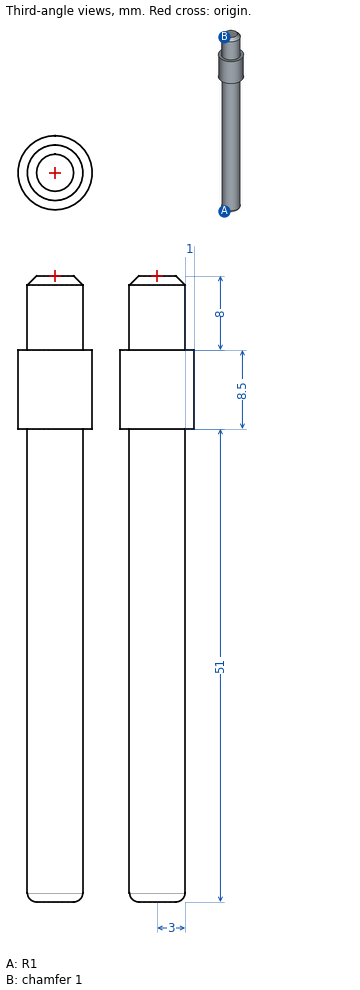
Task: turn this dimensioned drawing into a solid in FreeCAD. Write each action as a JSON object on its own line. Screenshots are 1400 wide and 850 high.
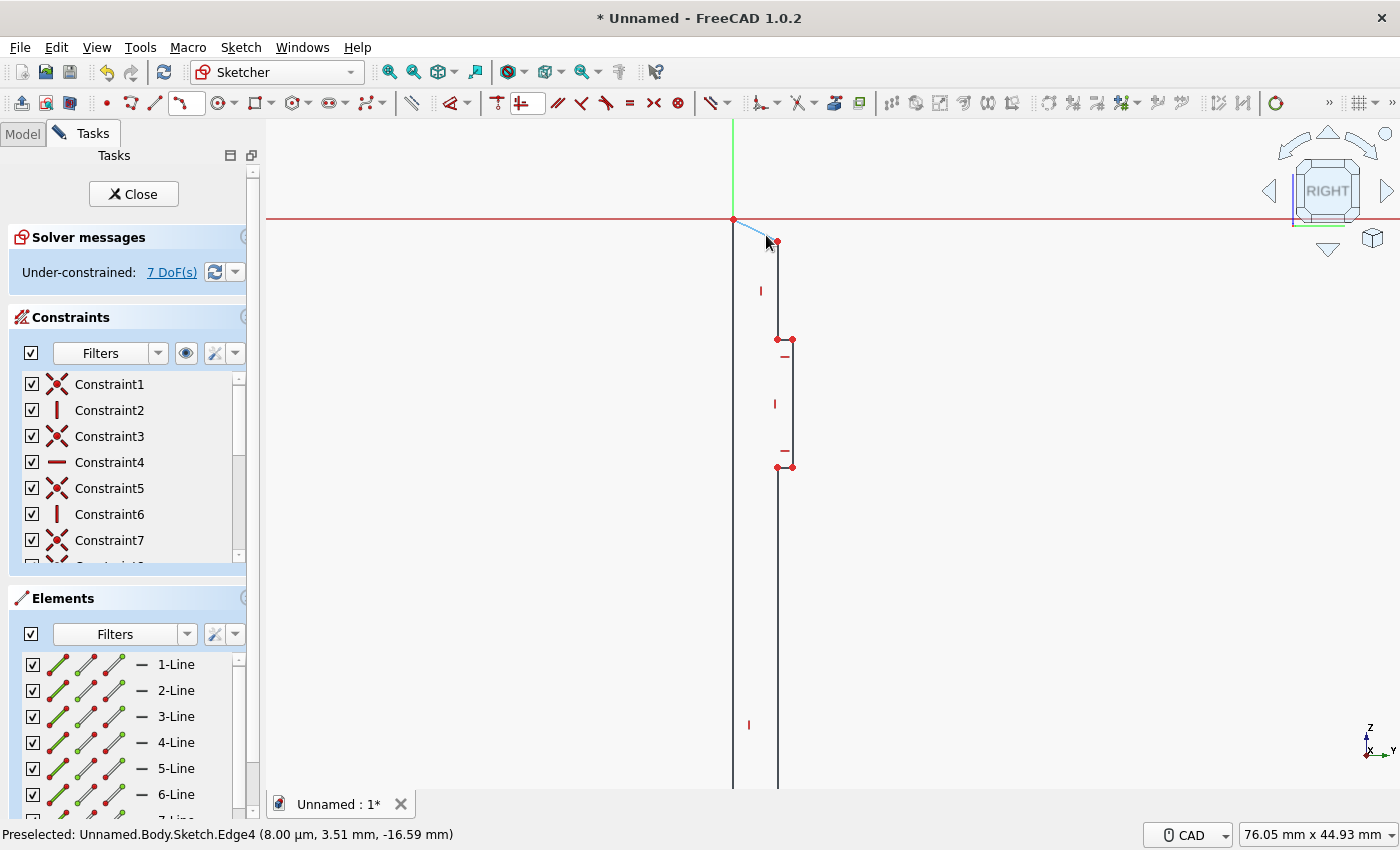
{"action": "left_click", "coordinate": [764, 235]}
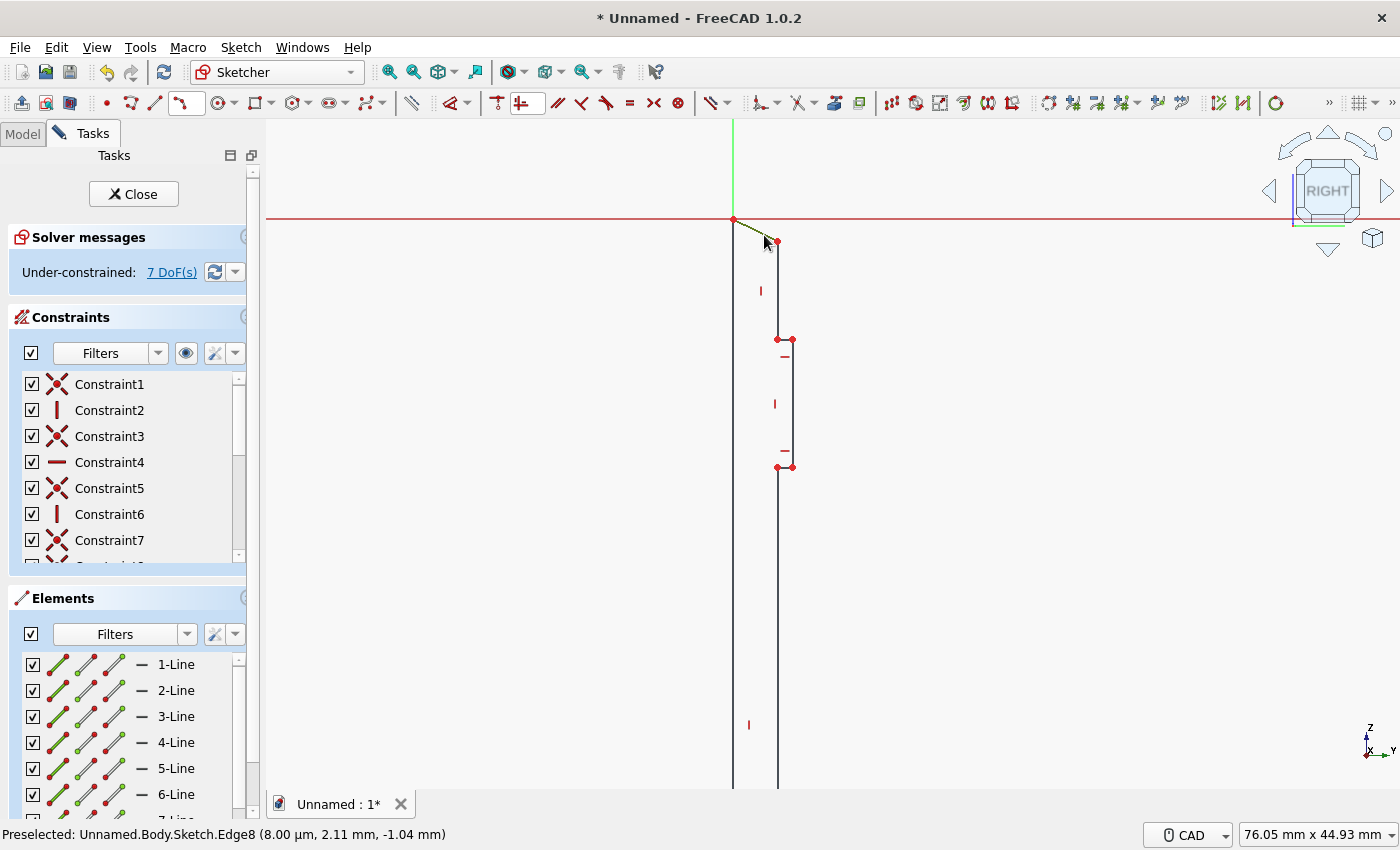
{"action": "key", "text": "h"}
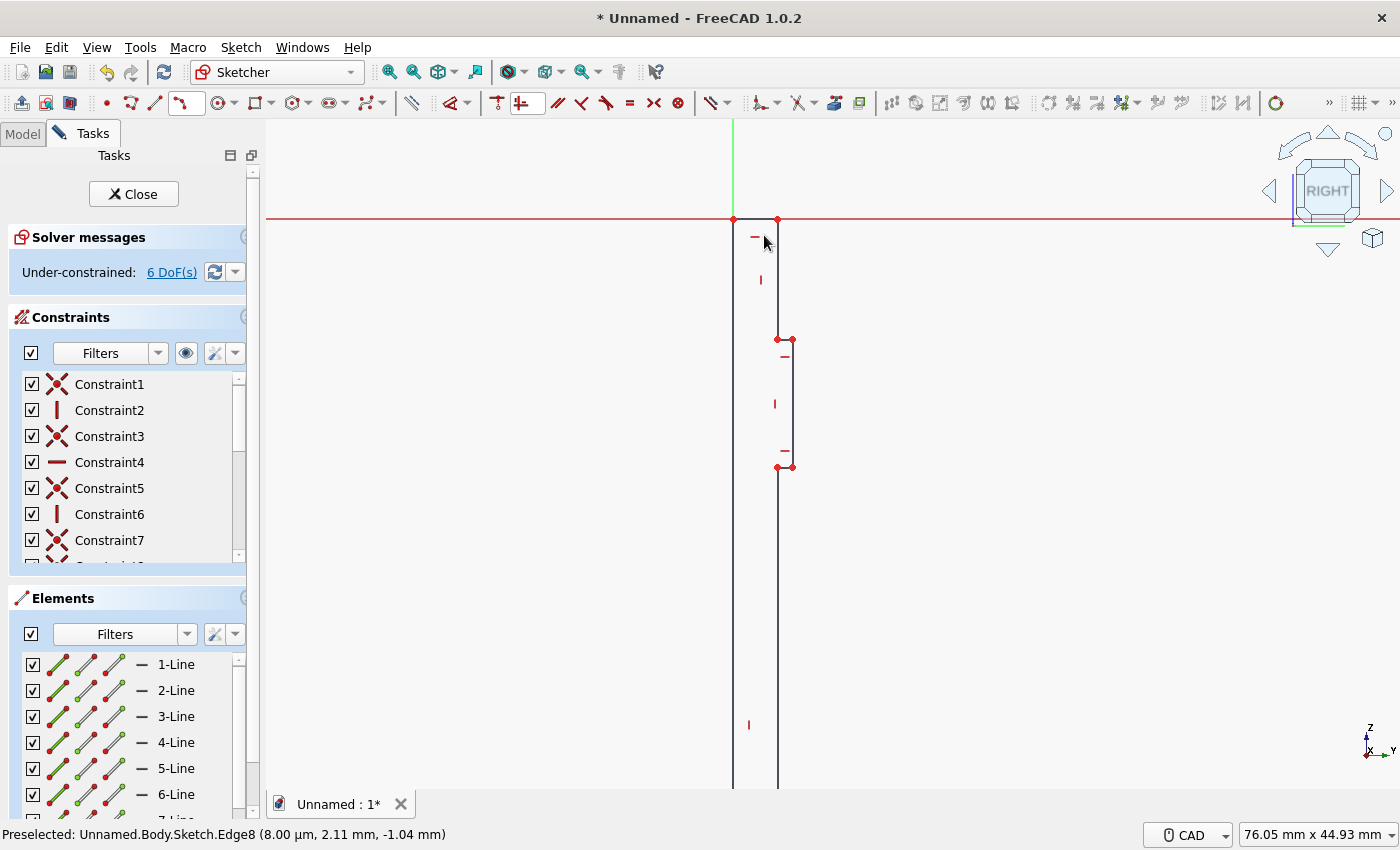
{"action": "key", "text": "d"}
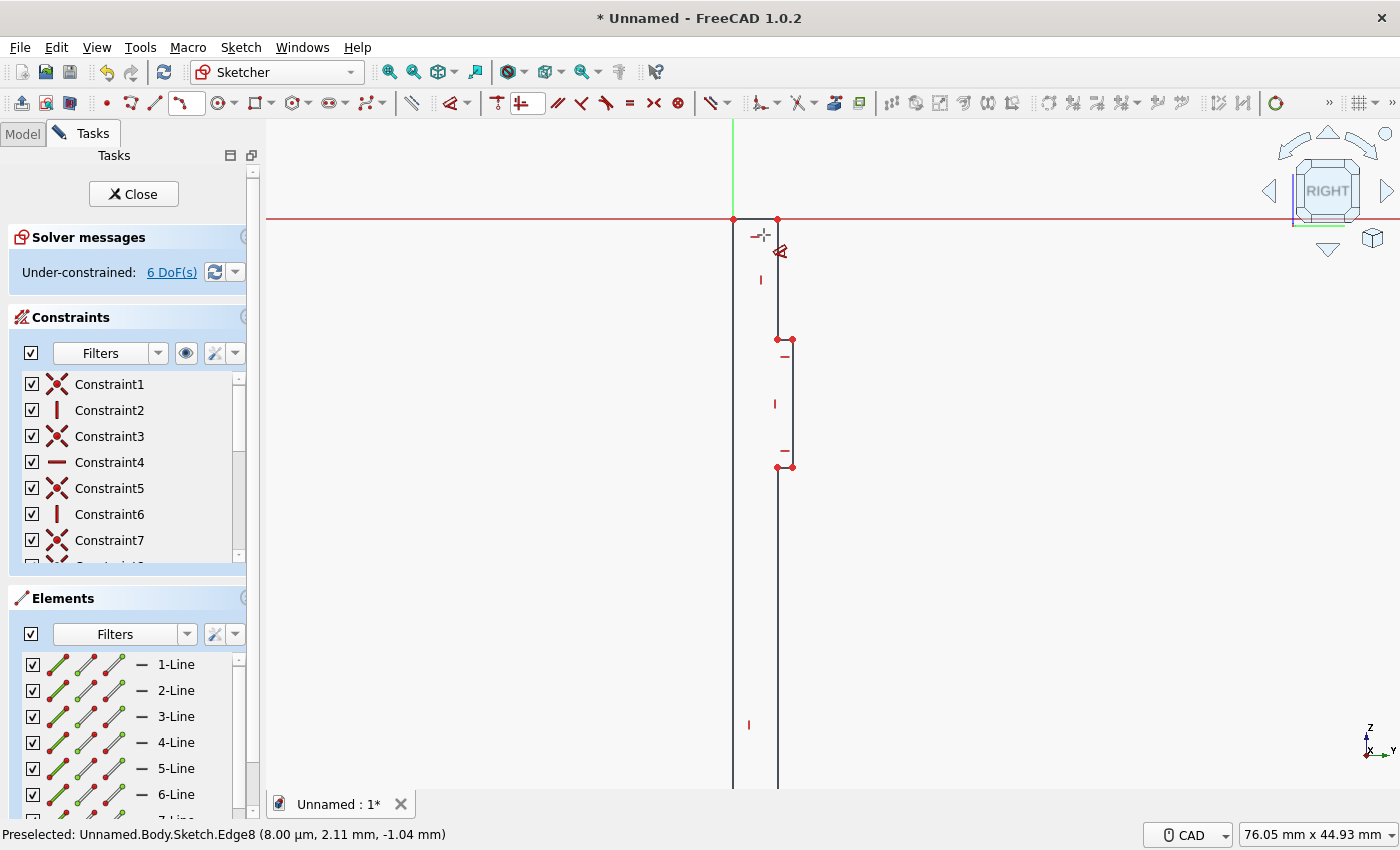
{"action": "scroll", "coordinate": [766, 235], "scroll_direction": "down", "scroll_amount": 4}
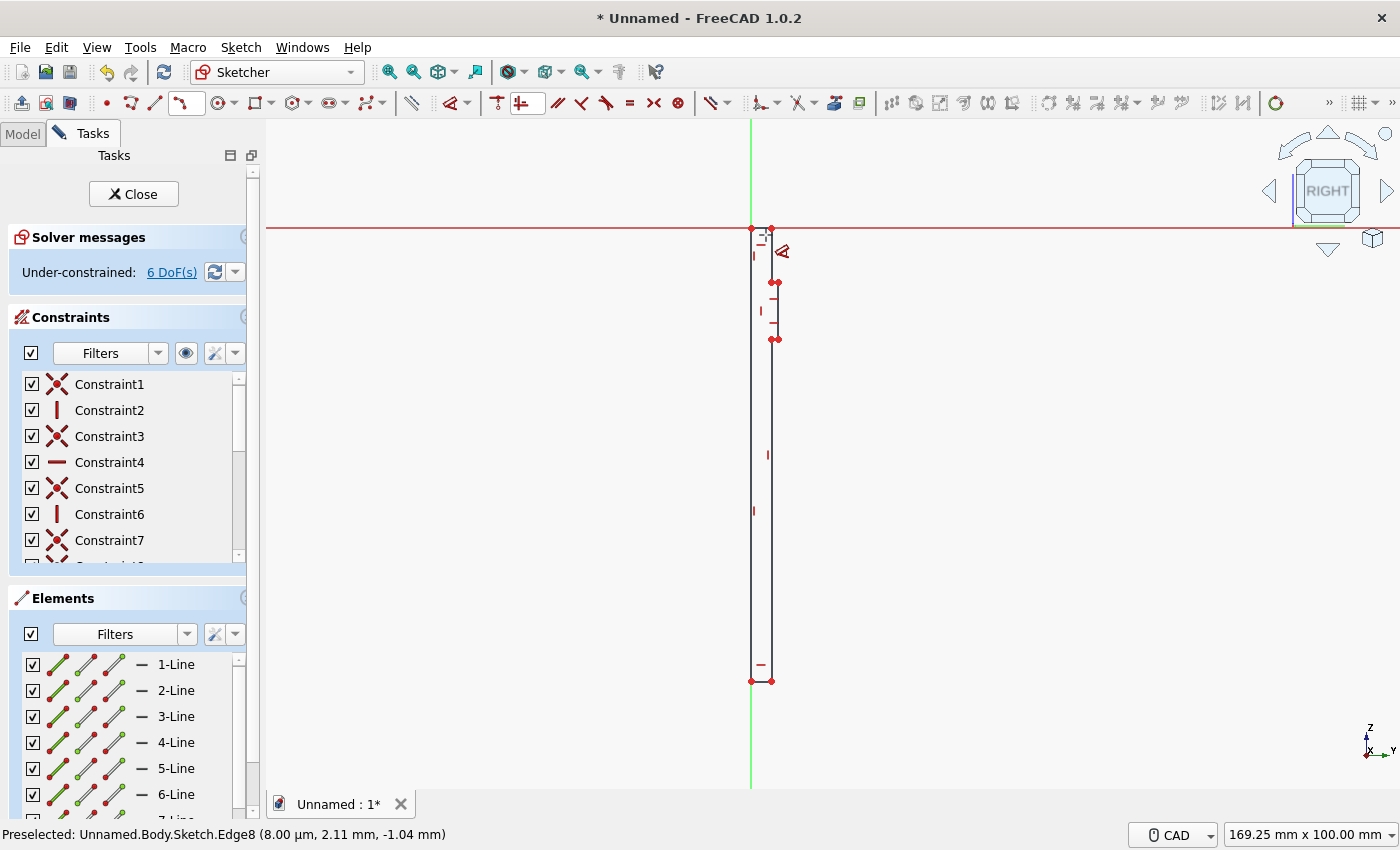
{"action": "scroll", "coordinate": [757, 682], "scroll_direction": "up", "scroll_amount": 5}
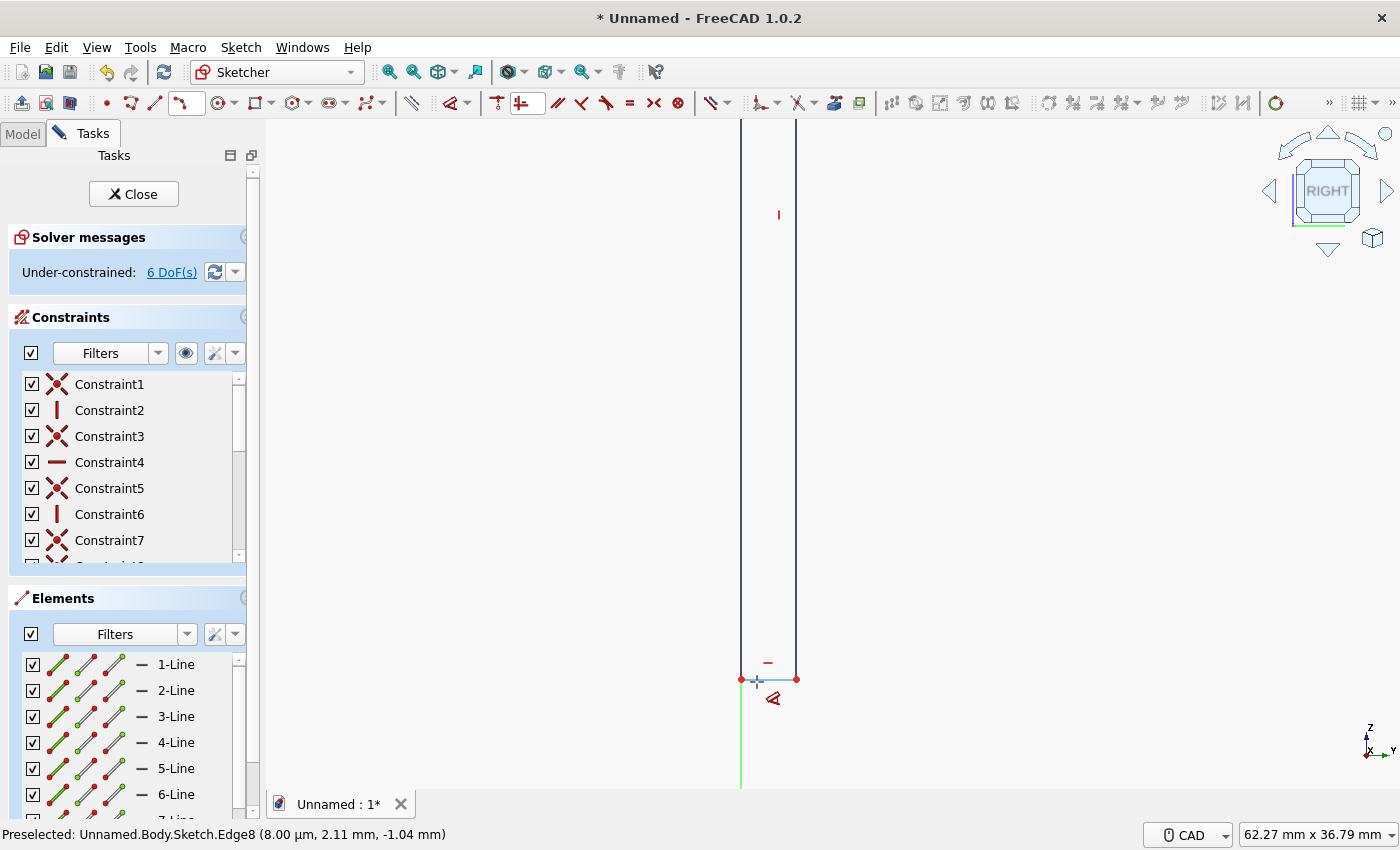
{"action": "left_click", "coordinate": [758, 680]}
{"action": "left_click", "coordinate": [769, 714]}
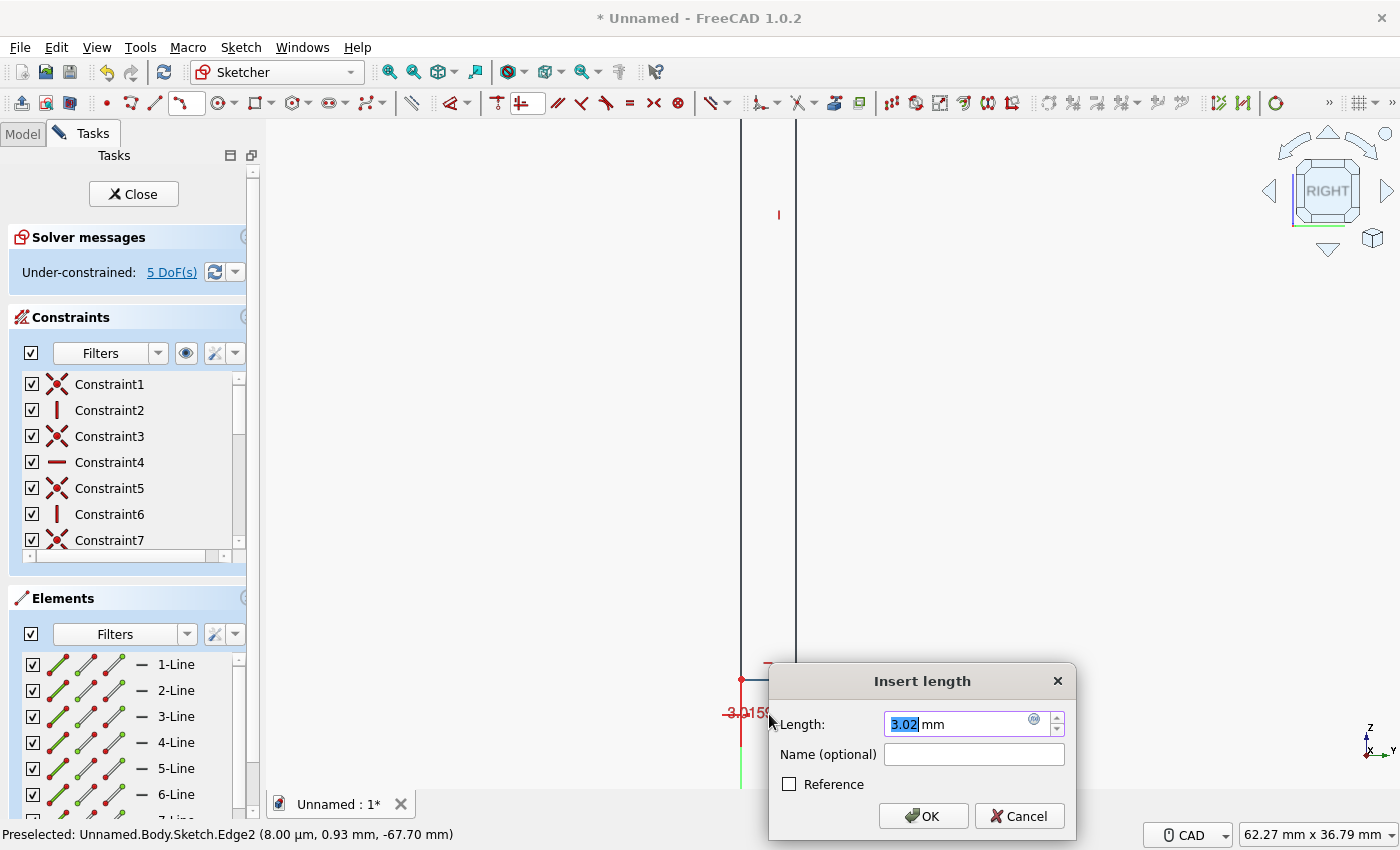
{"action": "type", "text": "3"}
{"action": "key", "text": "Return"}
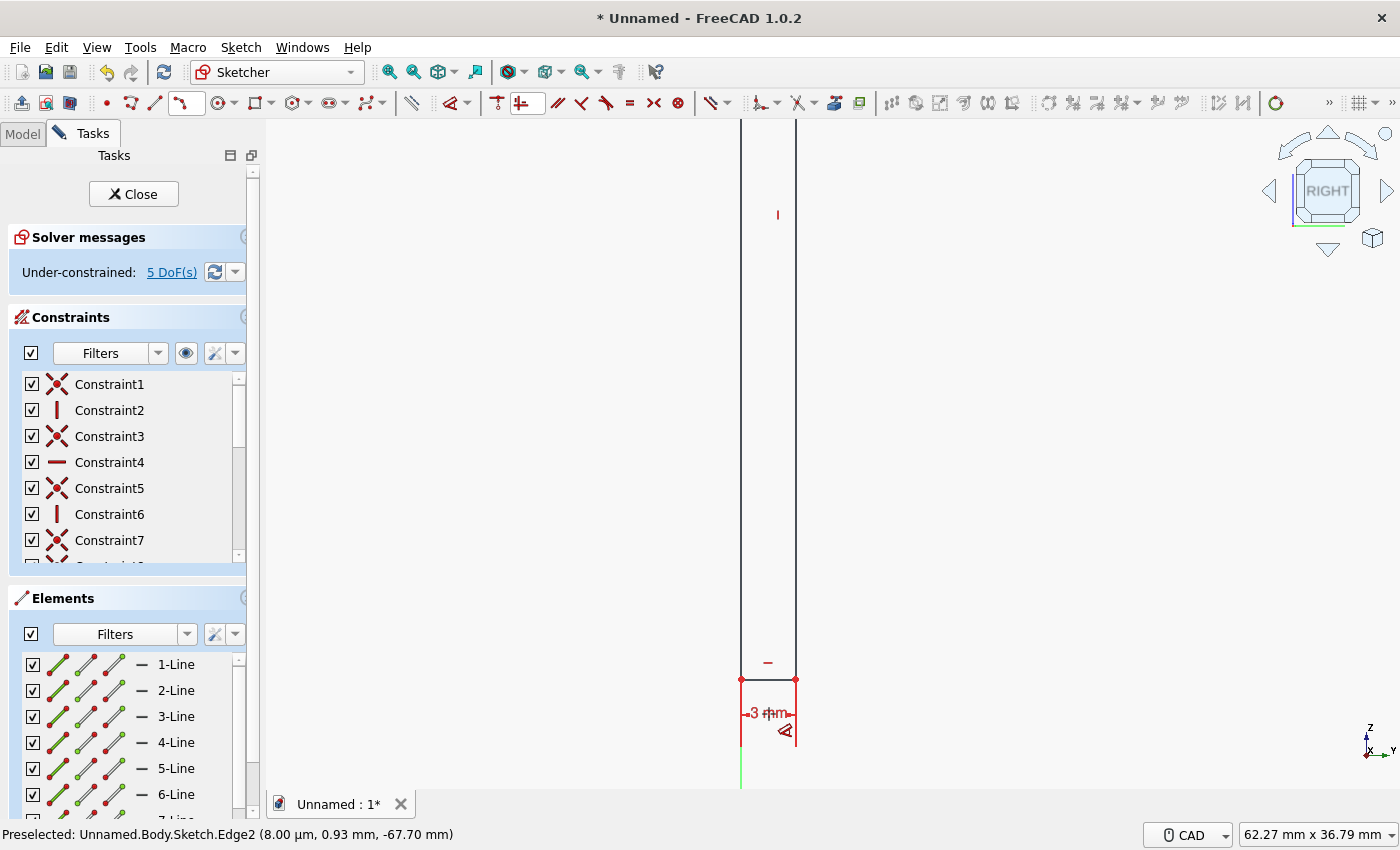
{"action": "scroll", "coordinate": [757, 683], "scroll_direction": "down", "scroll_amount": 5}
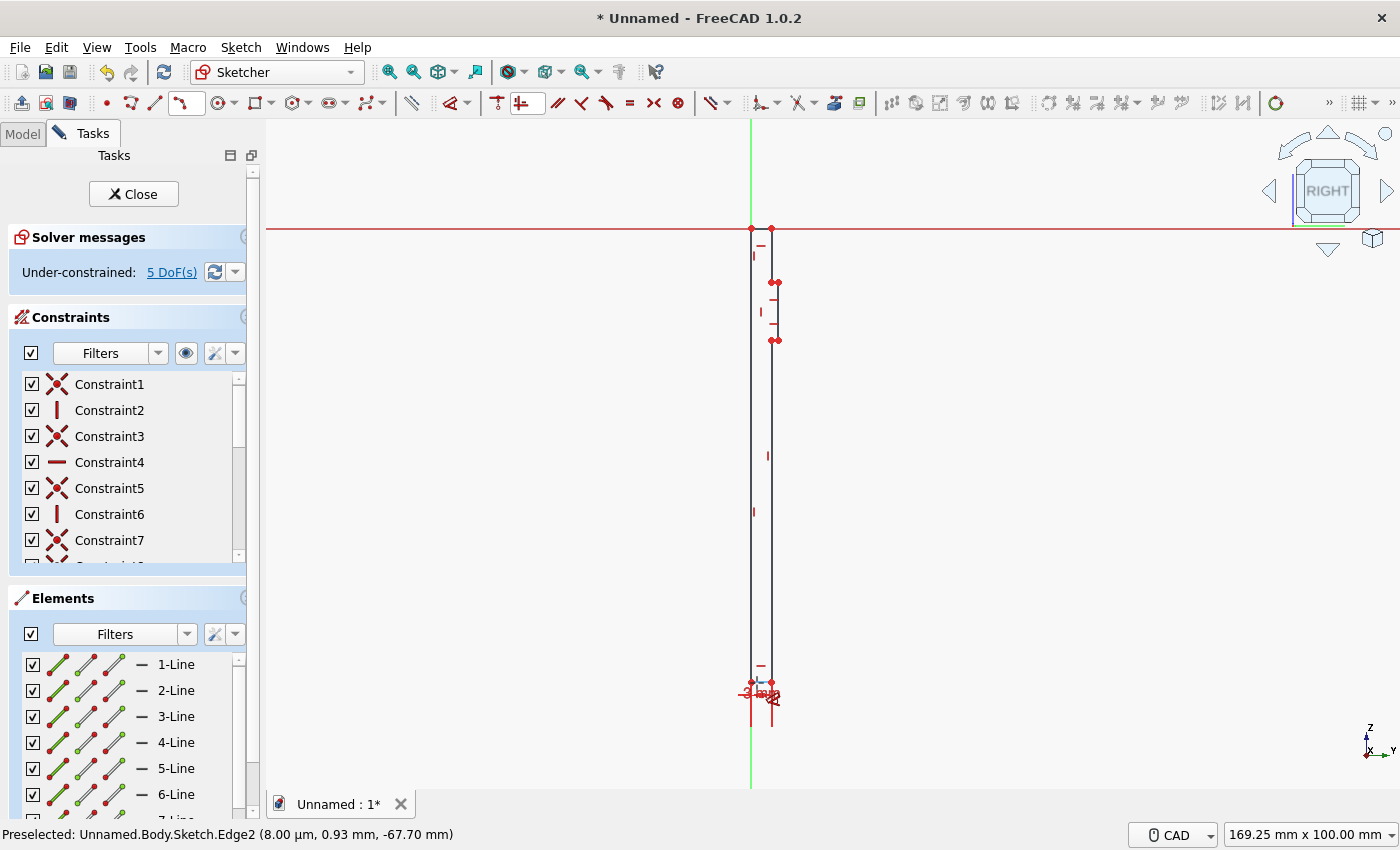
{"action": "scroll", "coordinate": [775, 340], "scroll_direction": "up", "scroll_amount": 9}